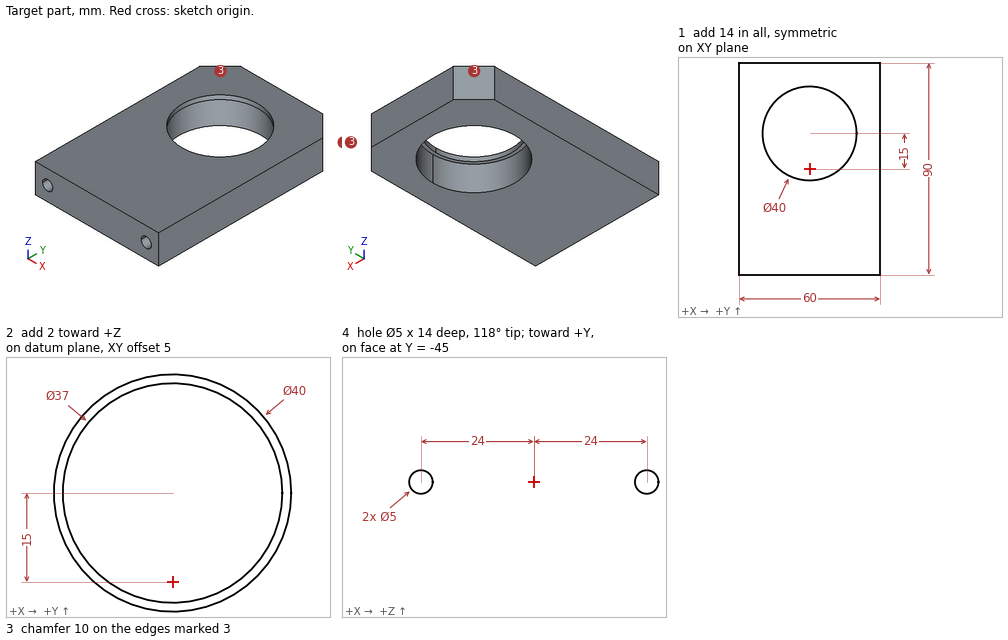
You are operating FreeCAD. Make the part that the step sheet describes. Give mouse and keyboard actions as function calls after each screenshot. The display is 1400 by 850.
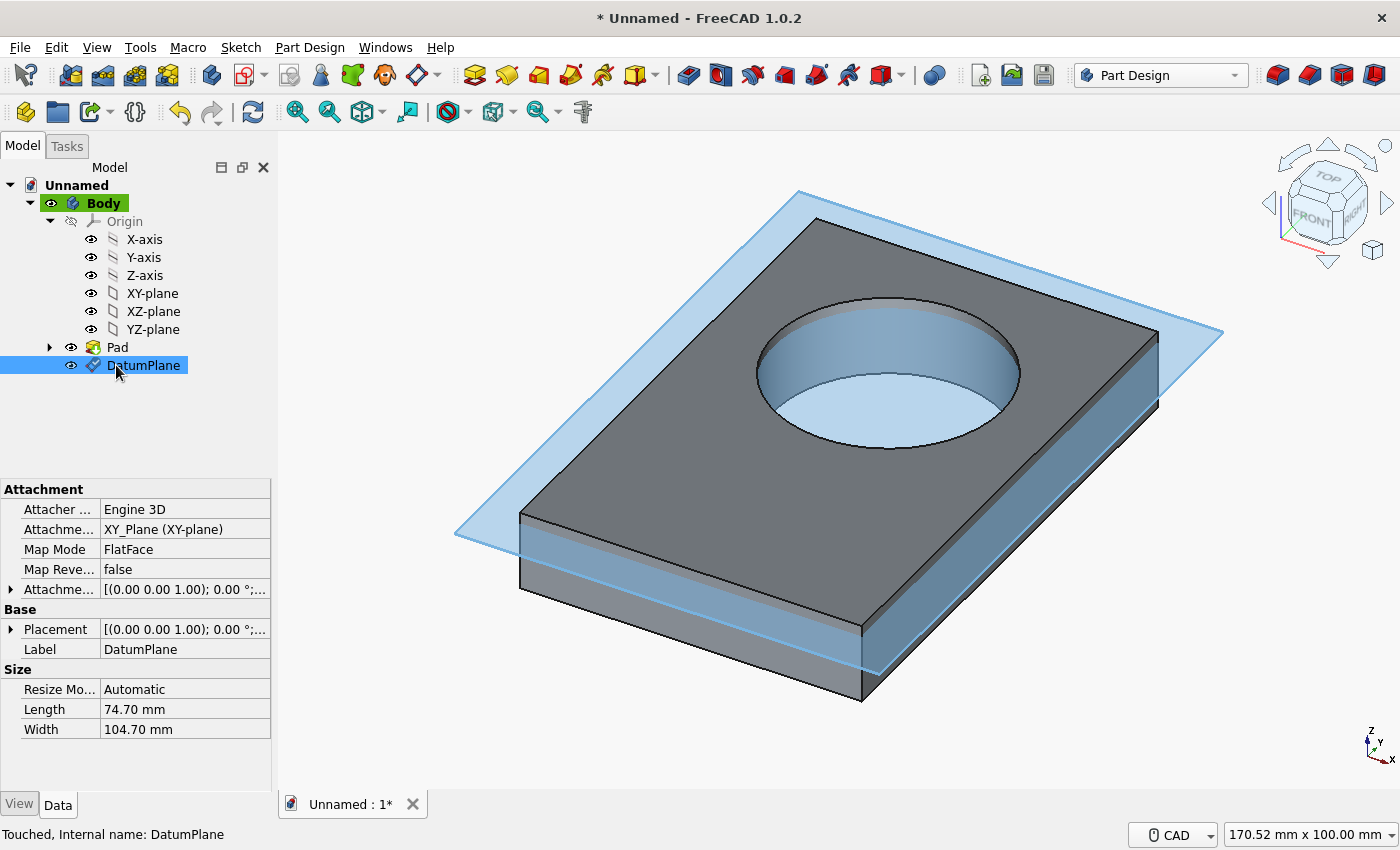
click(244, 76)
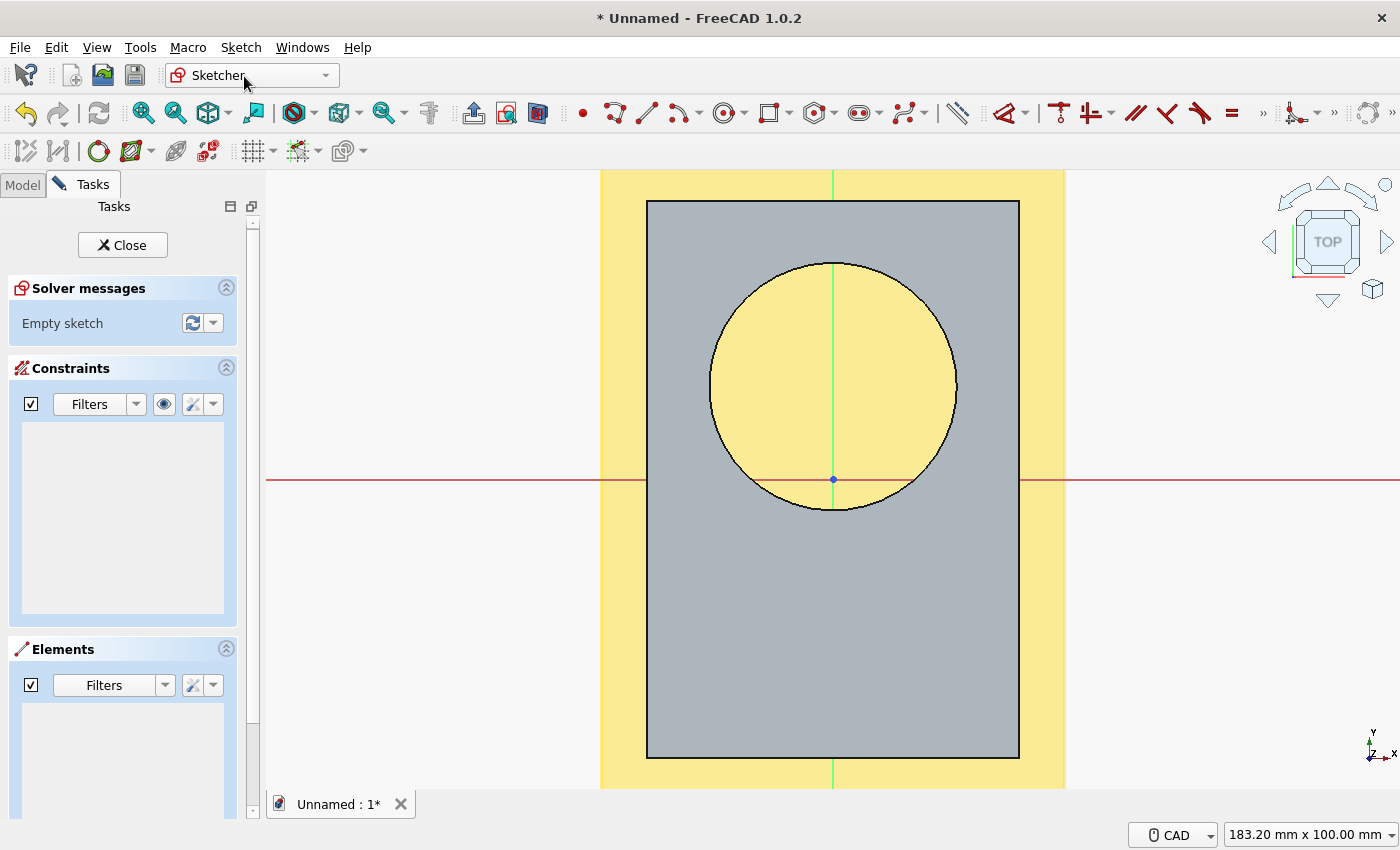
click(538, 114)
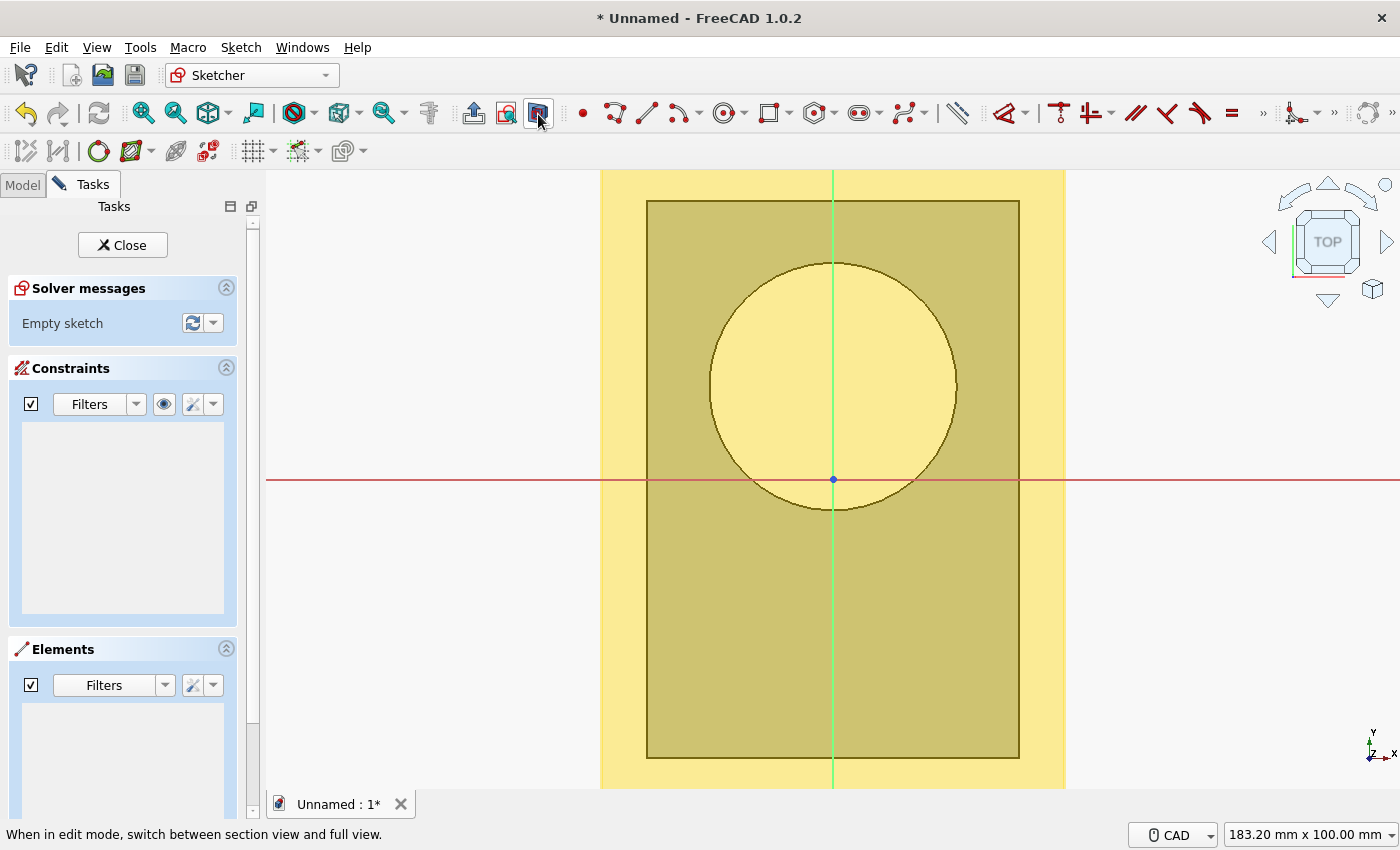
scroll(972, 198, up, 2)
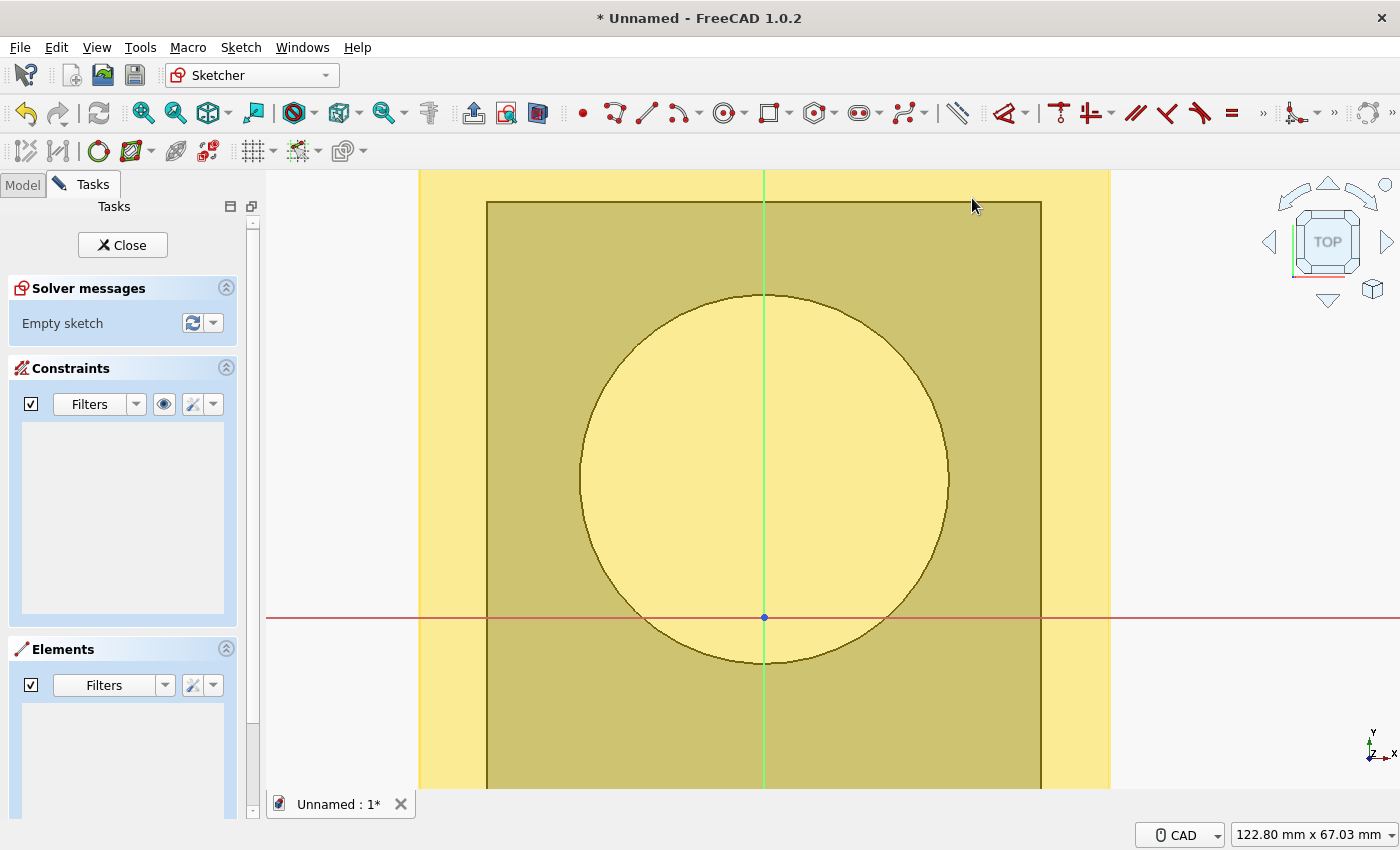
click(724, 114)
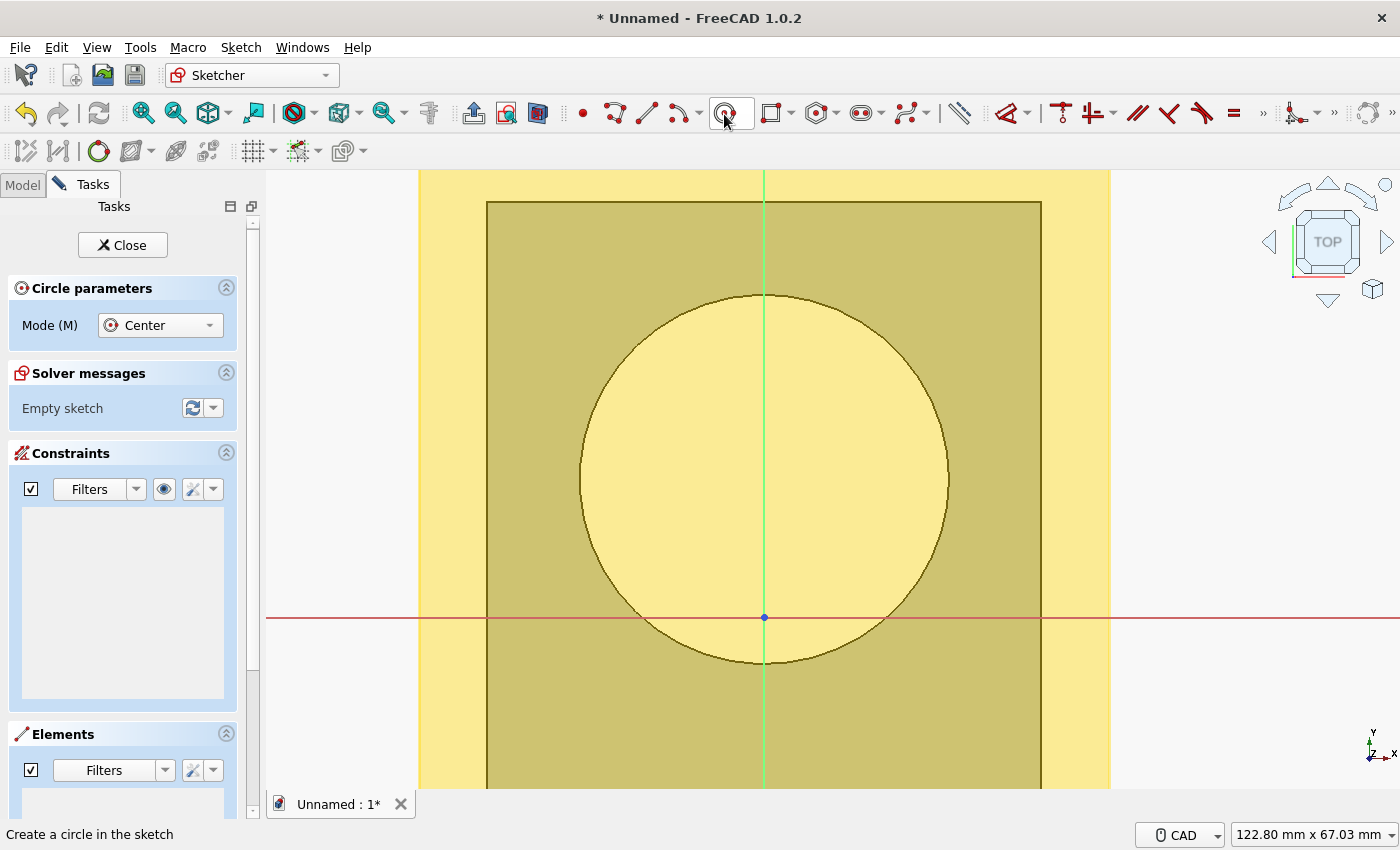
click(764, 479)
move(895, 349)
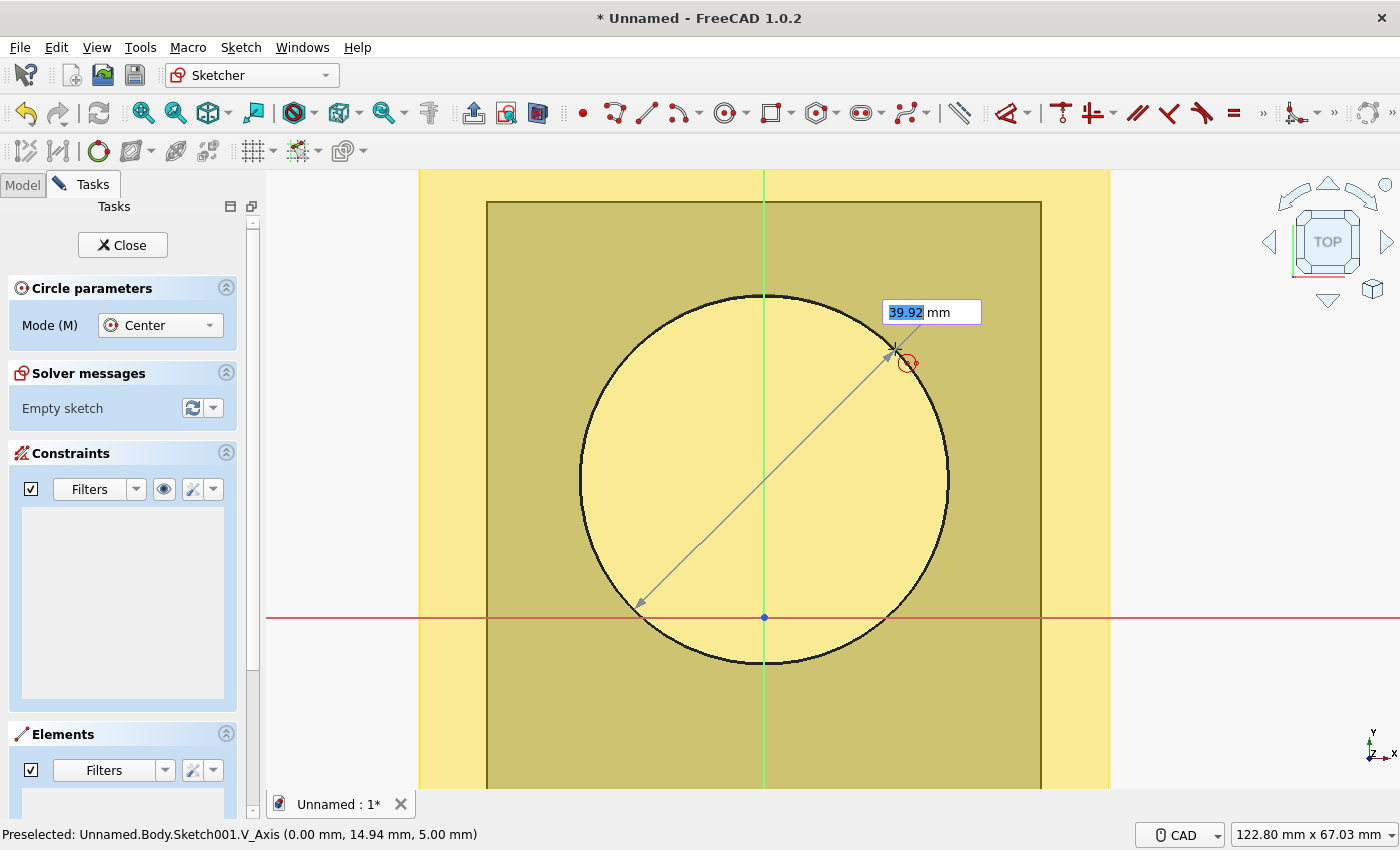
text(40)
key(Return)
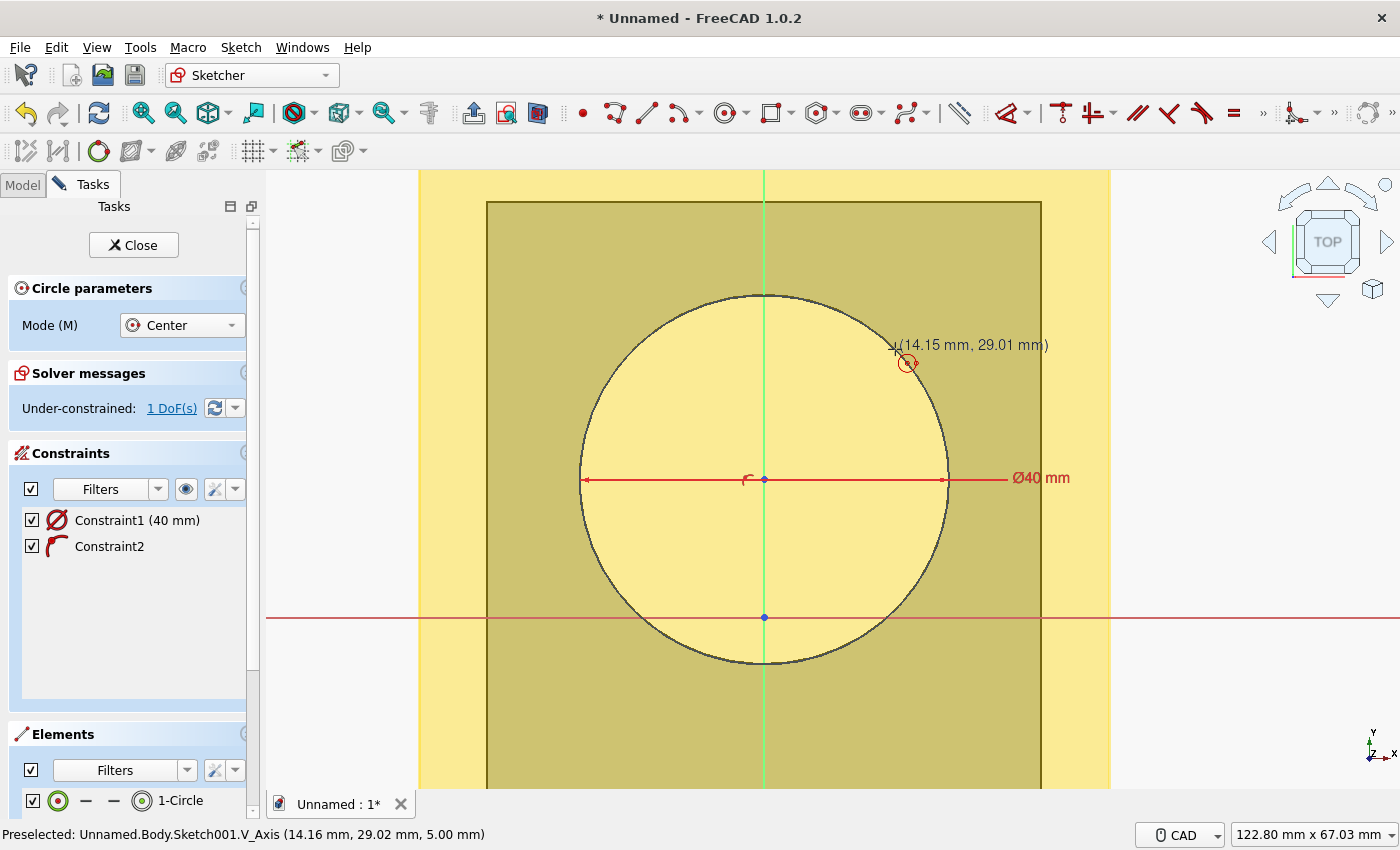
click(764, 480)
move(885, 359)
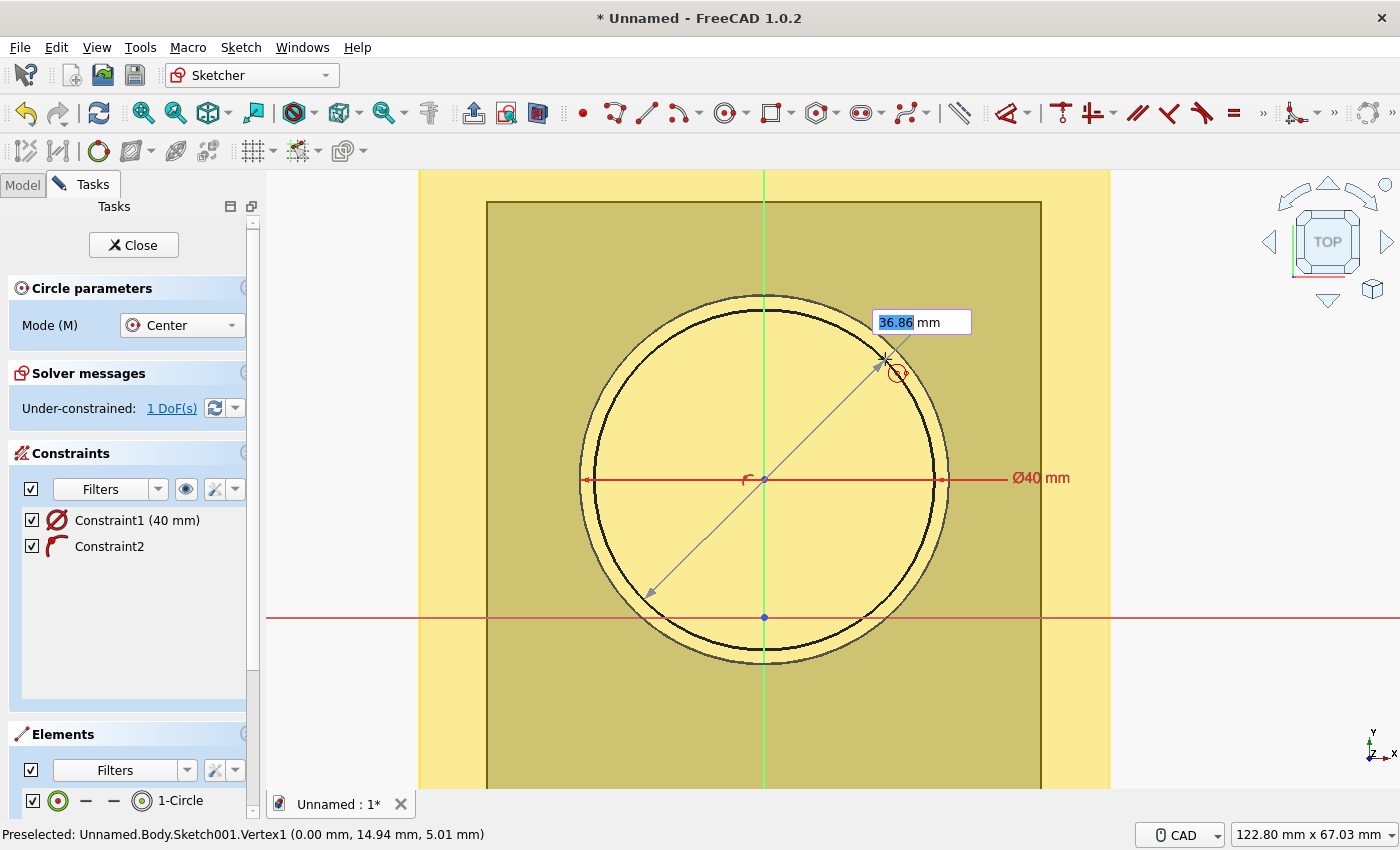
text(37)
key(Return)
key(Escape)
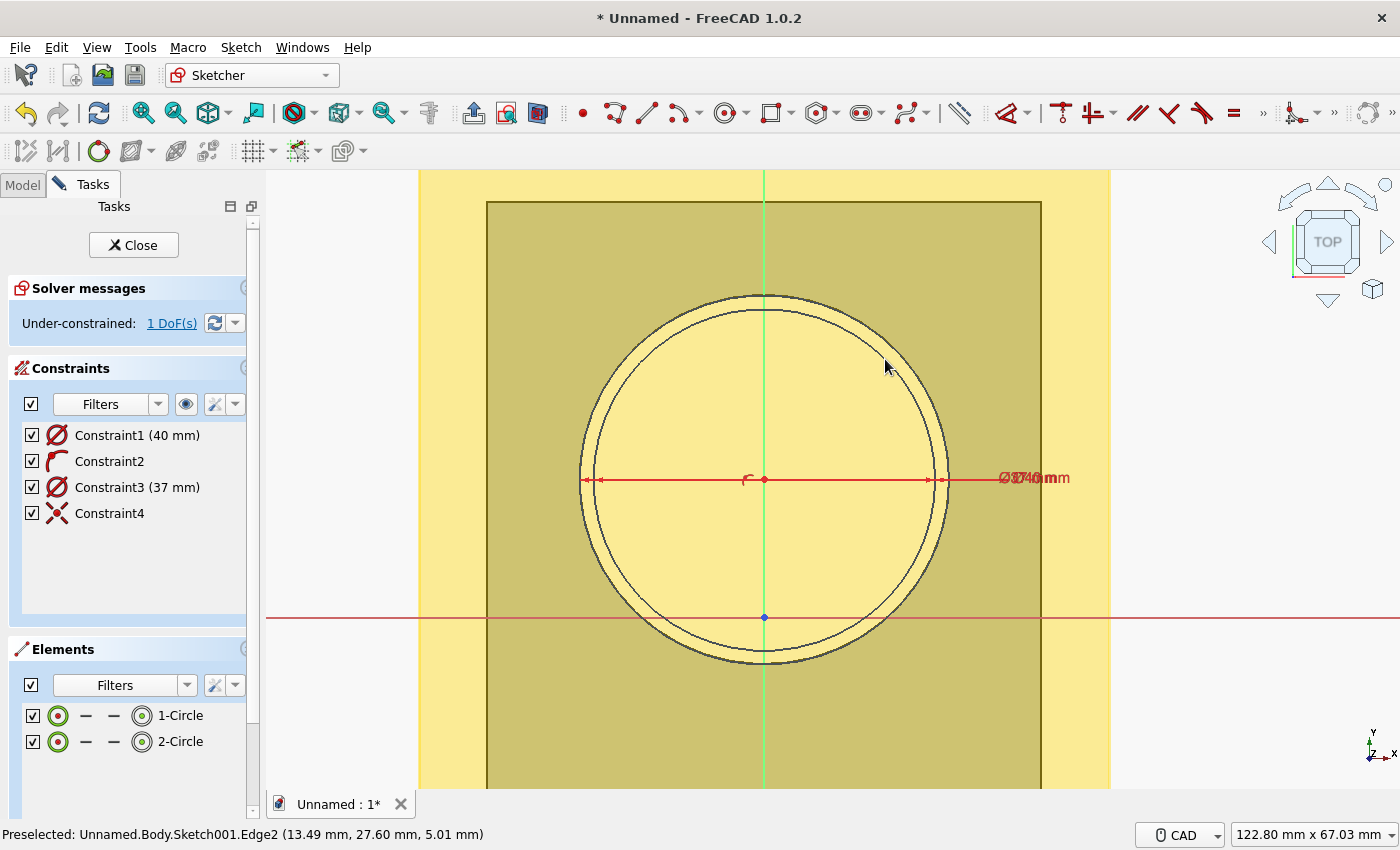
click(1006, 114)